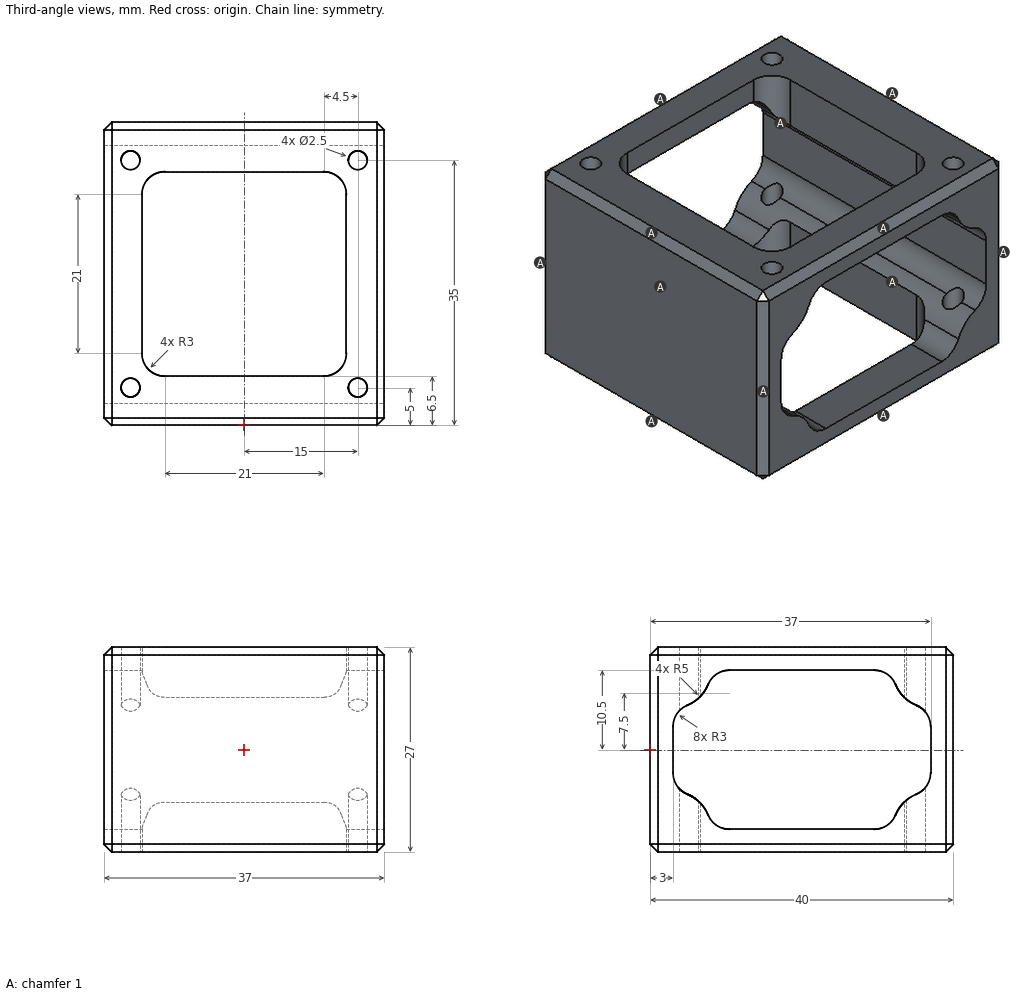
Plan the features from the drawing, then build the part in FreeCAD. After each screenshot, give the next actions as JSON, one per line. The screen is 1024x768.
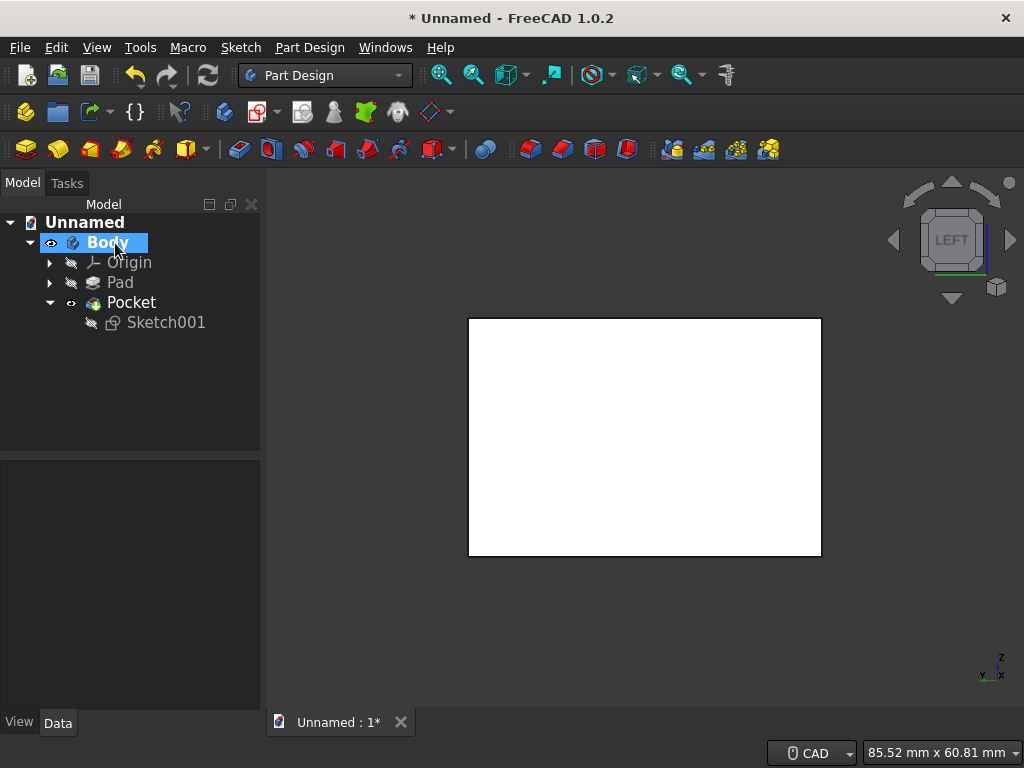
{"action": "left_click", "coordinate": [594, 437]}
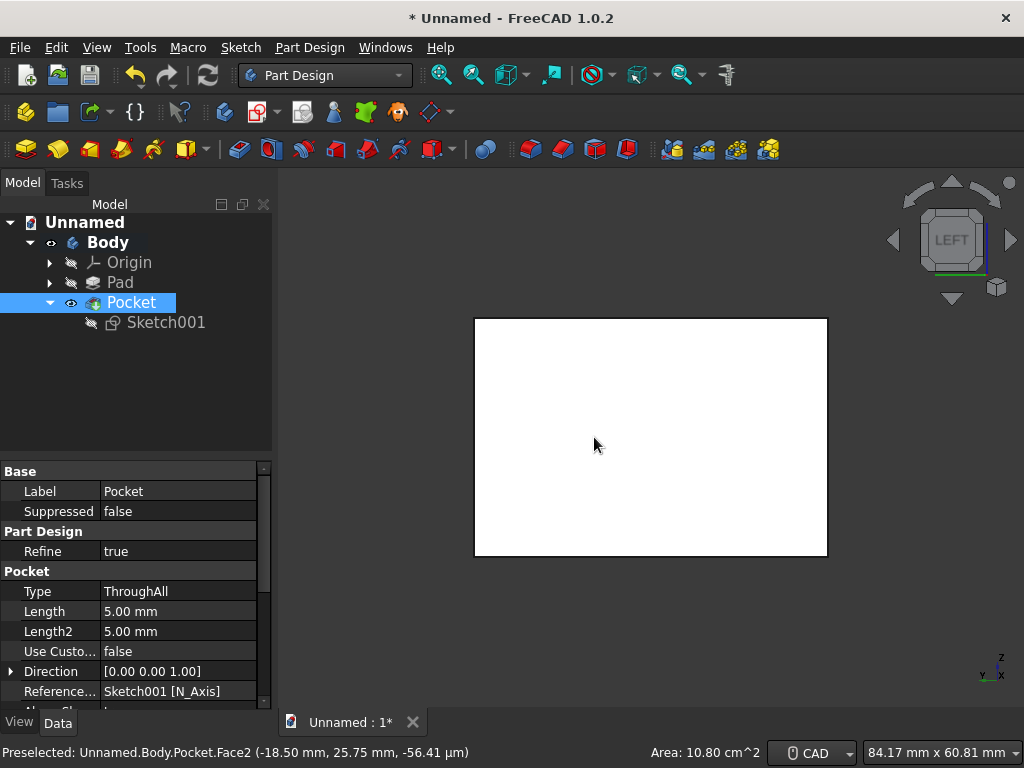
{"action": "left_click", "coordinate": [258, 112]}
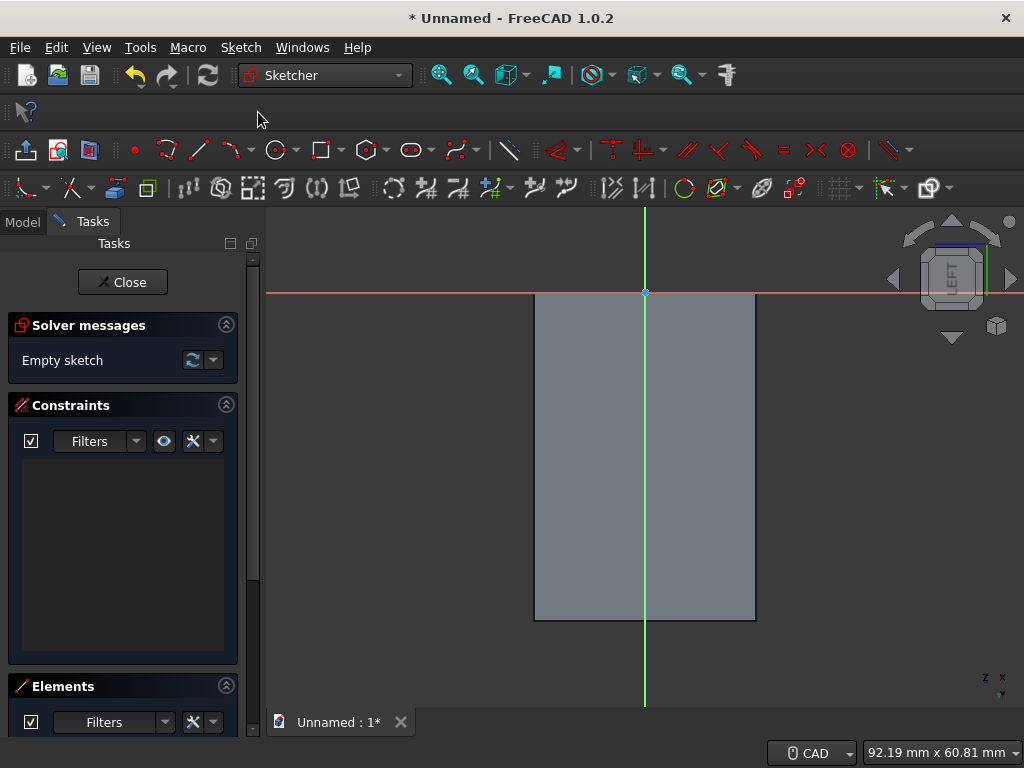
{"action": "left_click", "coordinate": [200, 150]}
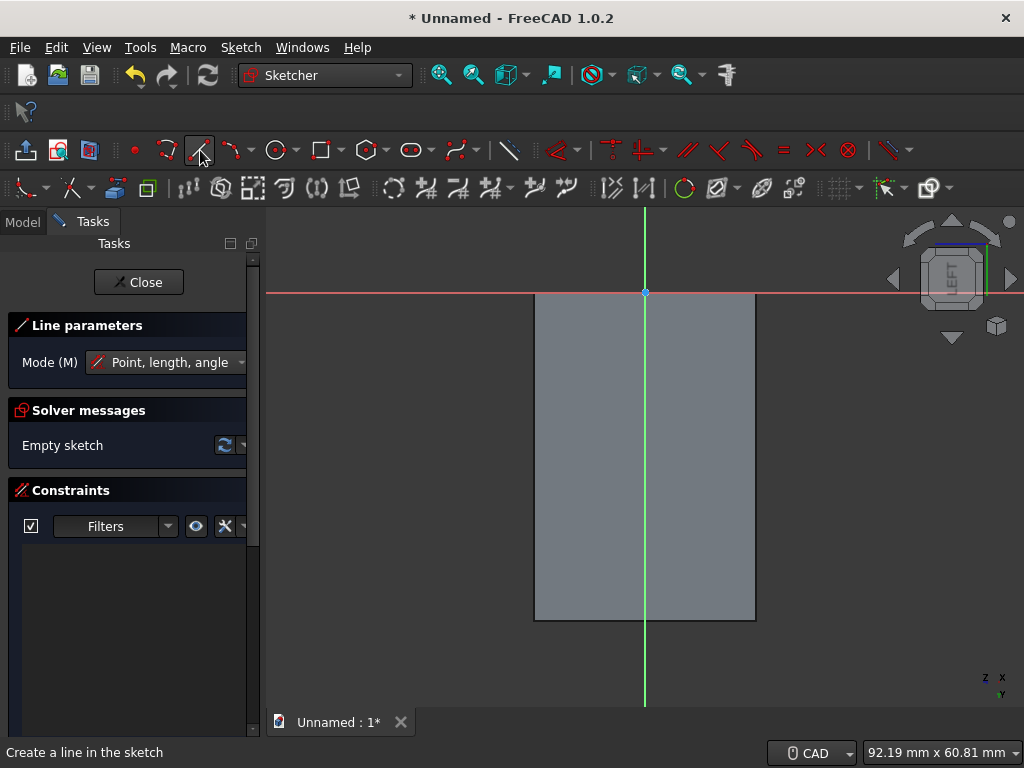
{"action": "left_click", "coordinate": [670, 317]}
{"action": "left_click", "coordinate": [620, 317]}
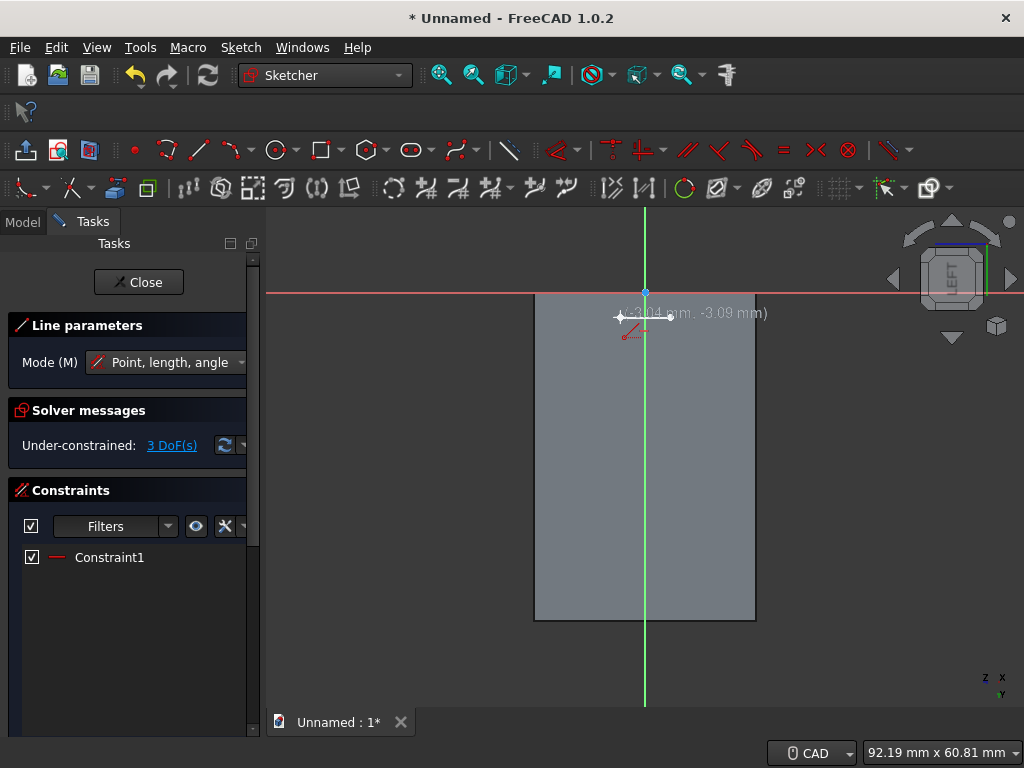
{"action": "left_click", "coordinate": [559, 378]}
{"action": "left_click", "coordinate": [559, 536]}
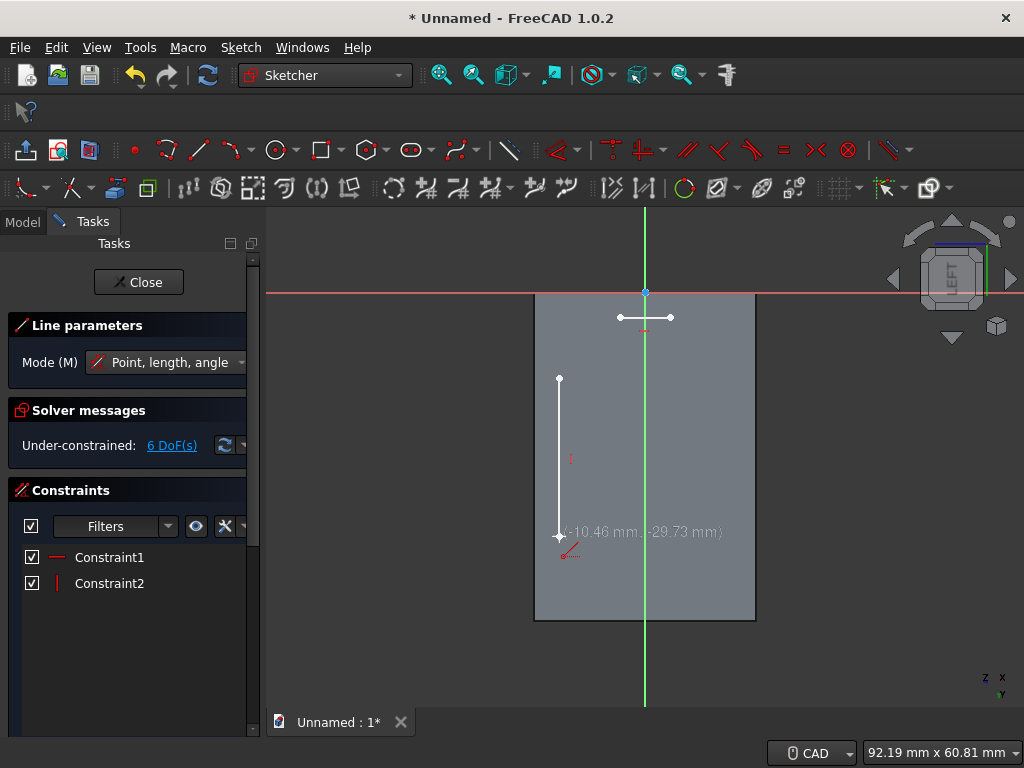
{"action": "left_click", "coordinate": [620, 597]}
{"action": "left_click", "coordinate": [670, 597]}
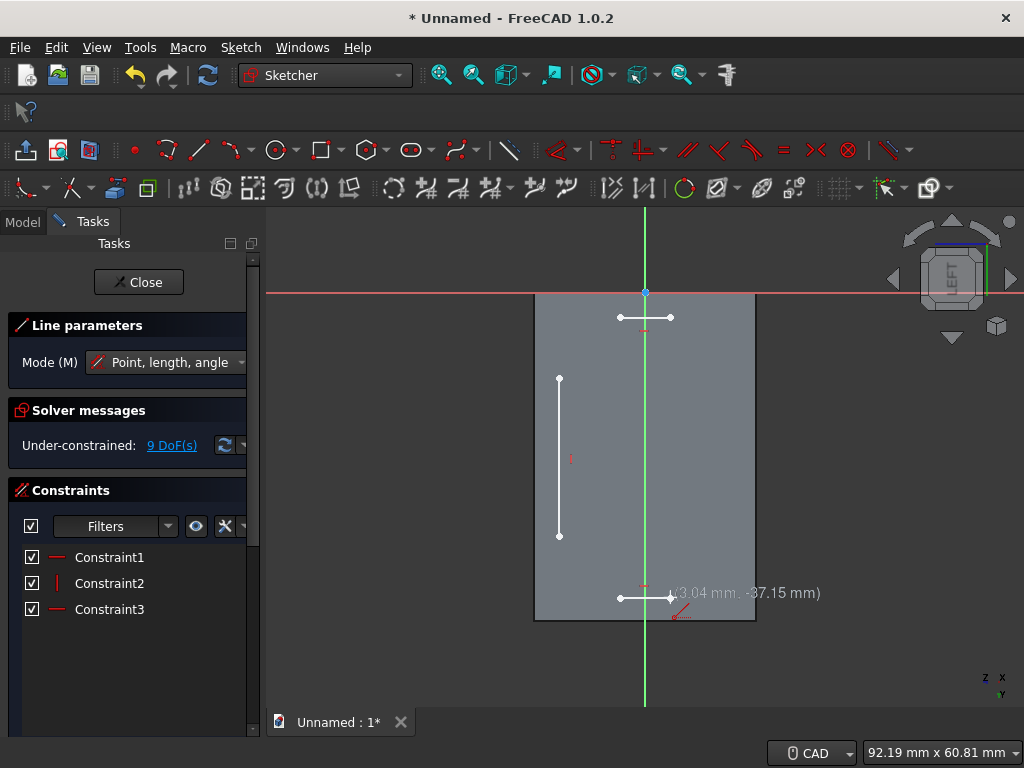
{"action": "left_click", "coordinate": [731, 536]}
{"action": "left_click", "coordinate": [731, 378]}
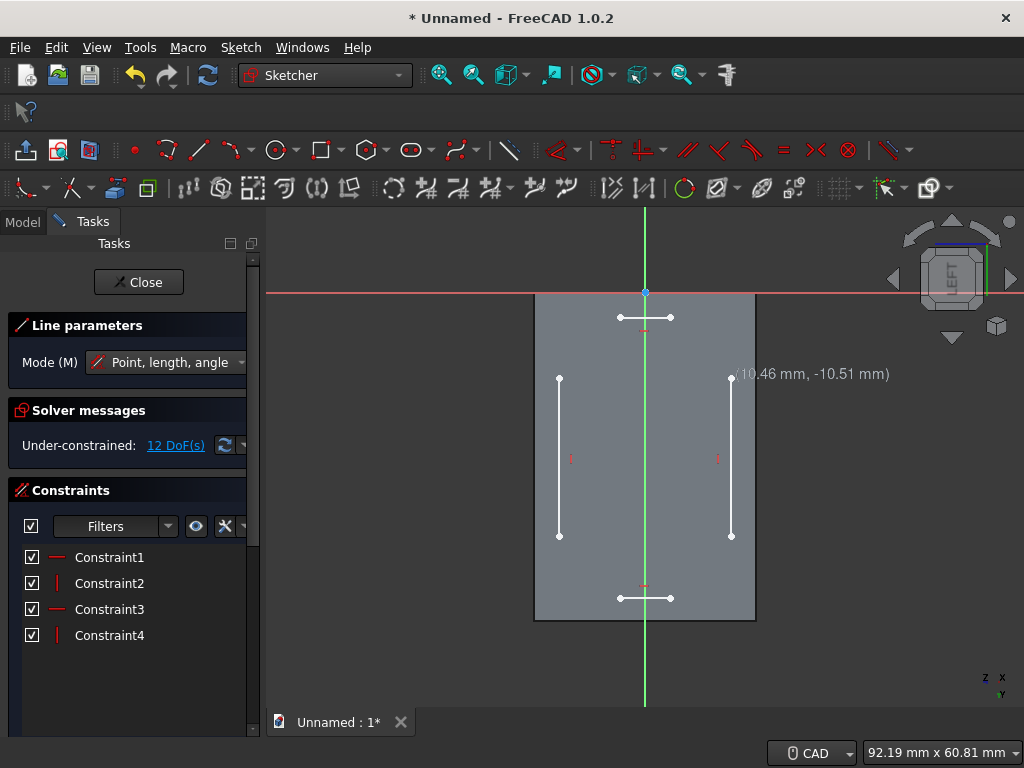
{"action": "left_click", "coordinate": [232, 150]}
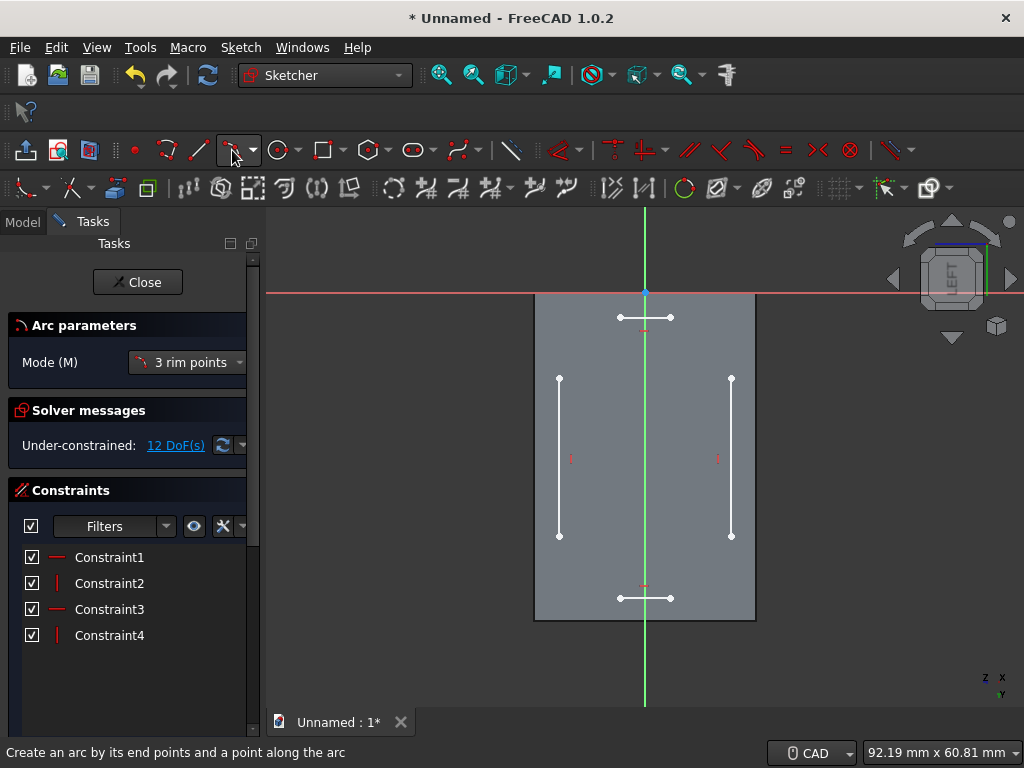
{"action": "left_click", "coordinate": [620, 318]}
{"action": "left_click", "coordinate": [597, 333]}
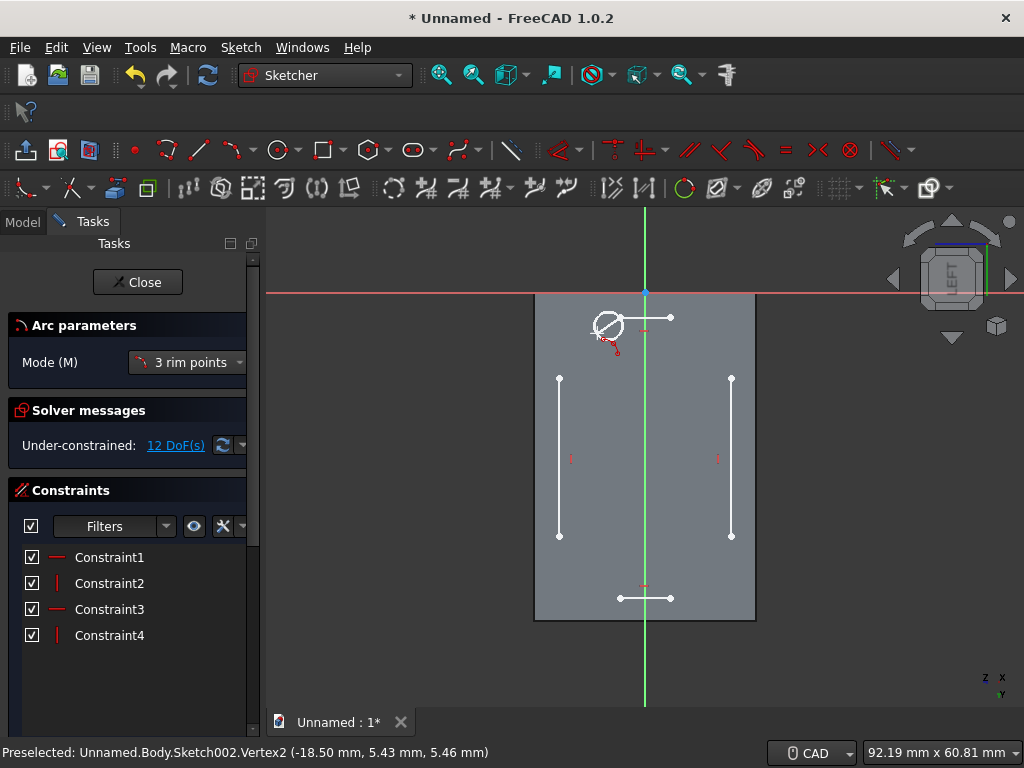
{"action": "scroll", "coordinate": [606, 321], "scroll_direction": "up", "scroll_amount": 7}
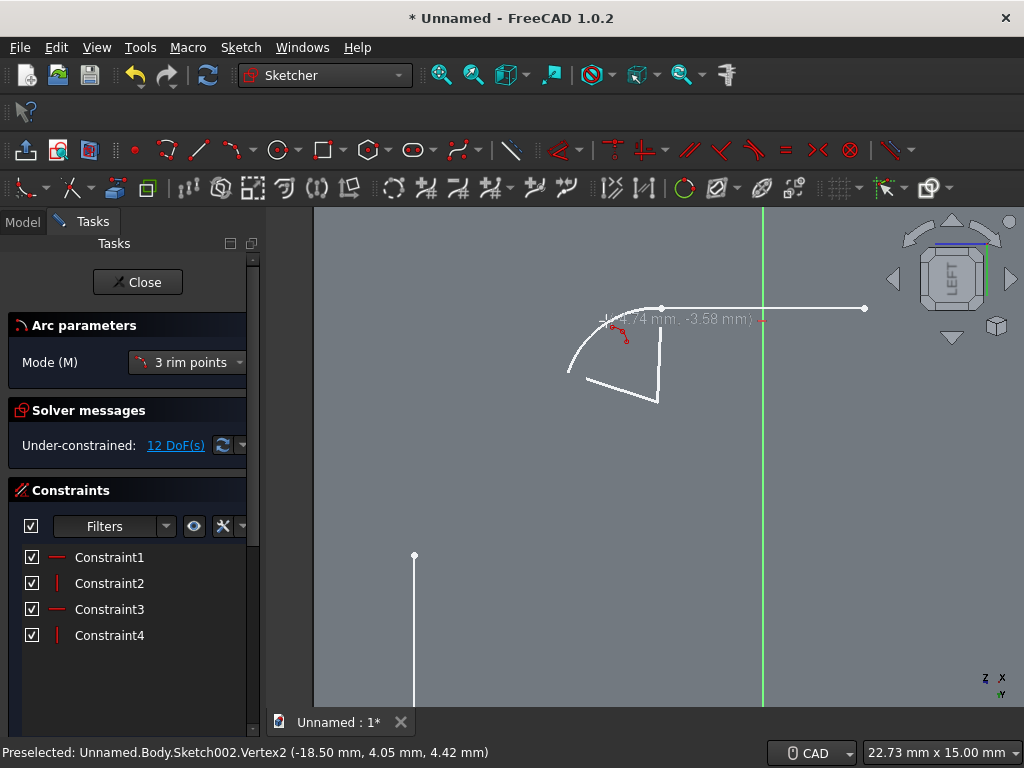
{"action": "left_click", "coordinate": [604, 322]}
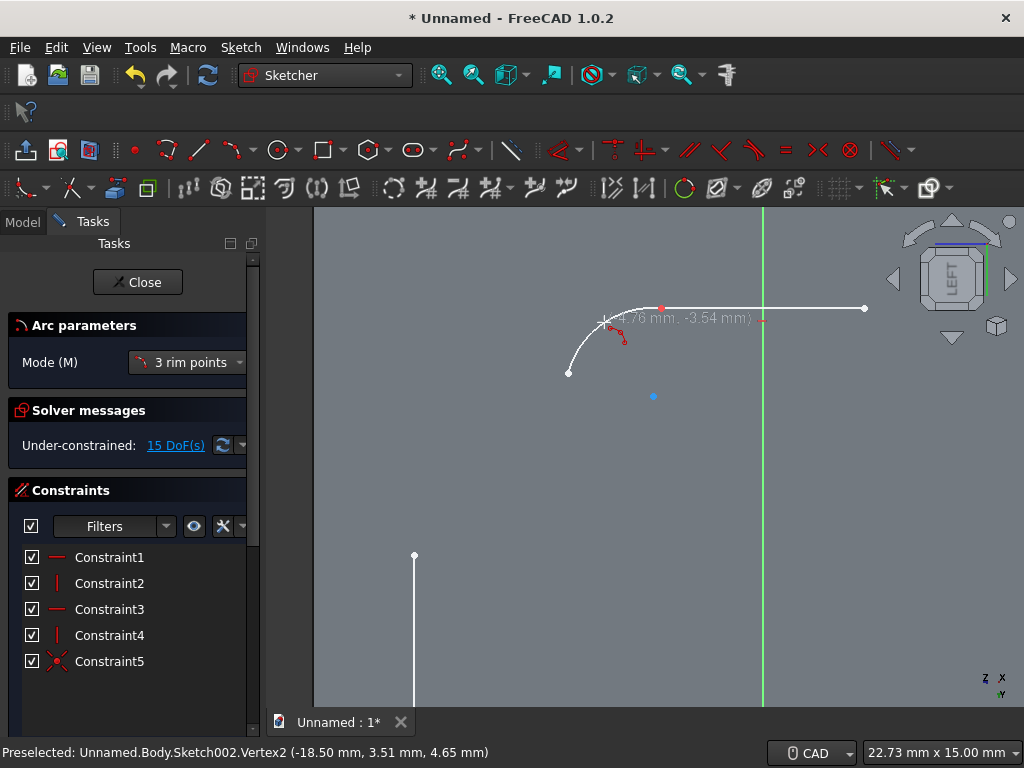
{"action": "scroll", "coordinate": [516, 338], "scroll_direction": "down", "scroll_amount": 7}